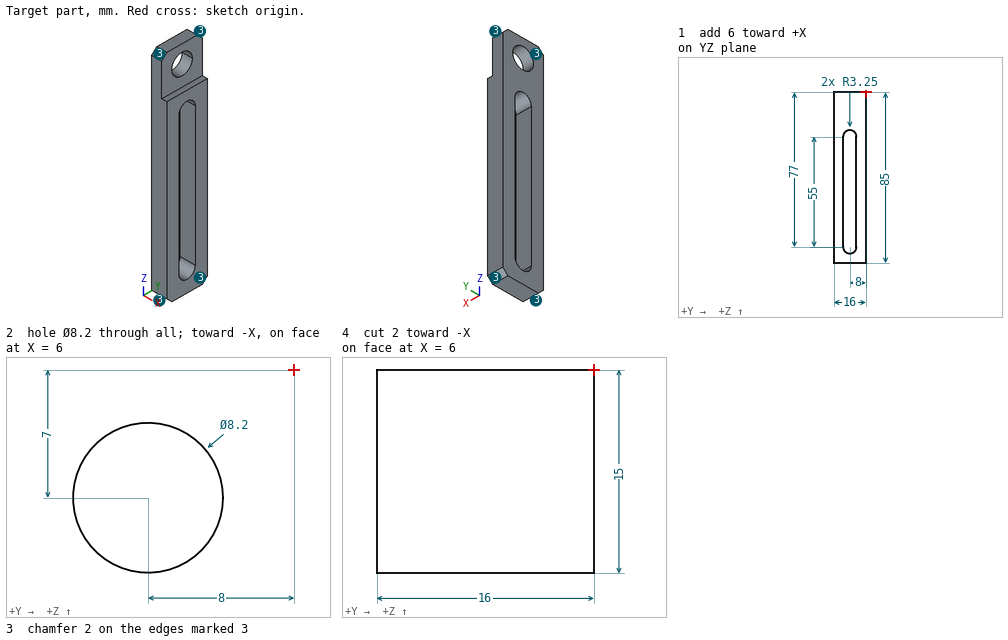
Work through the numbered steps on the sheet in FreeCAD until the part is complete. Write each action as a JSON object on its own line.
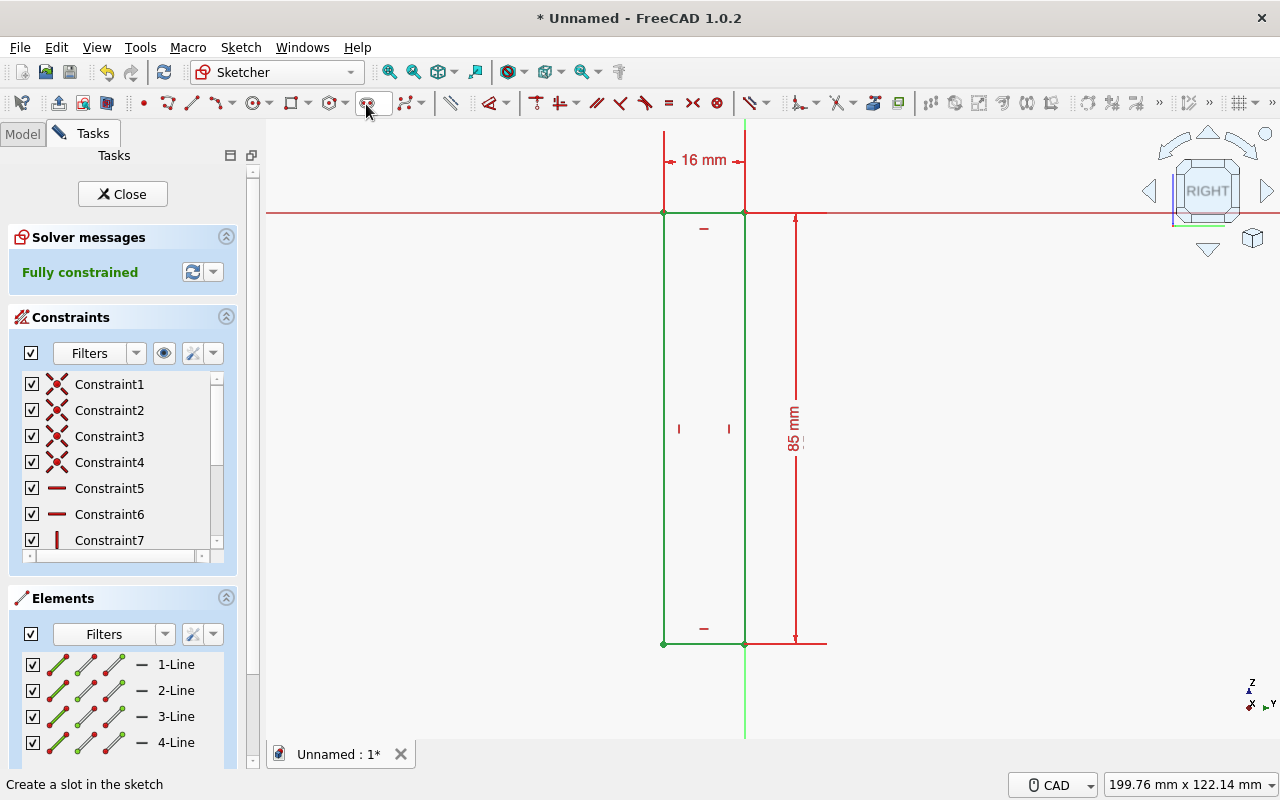
{"action": "scroll", "coordinate": [704, 604], "scroll_direction": "up", "scroll_amount": 2}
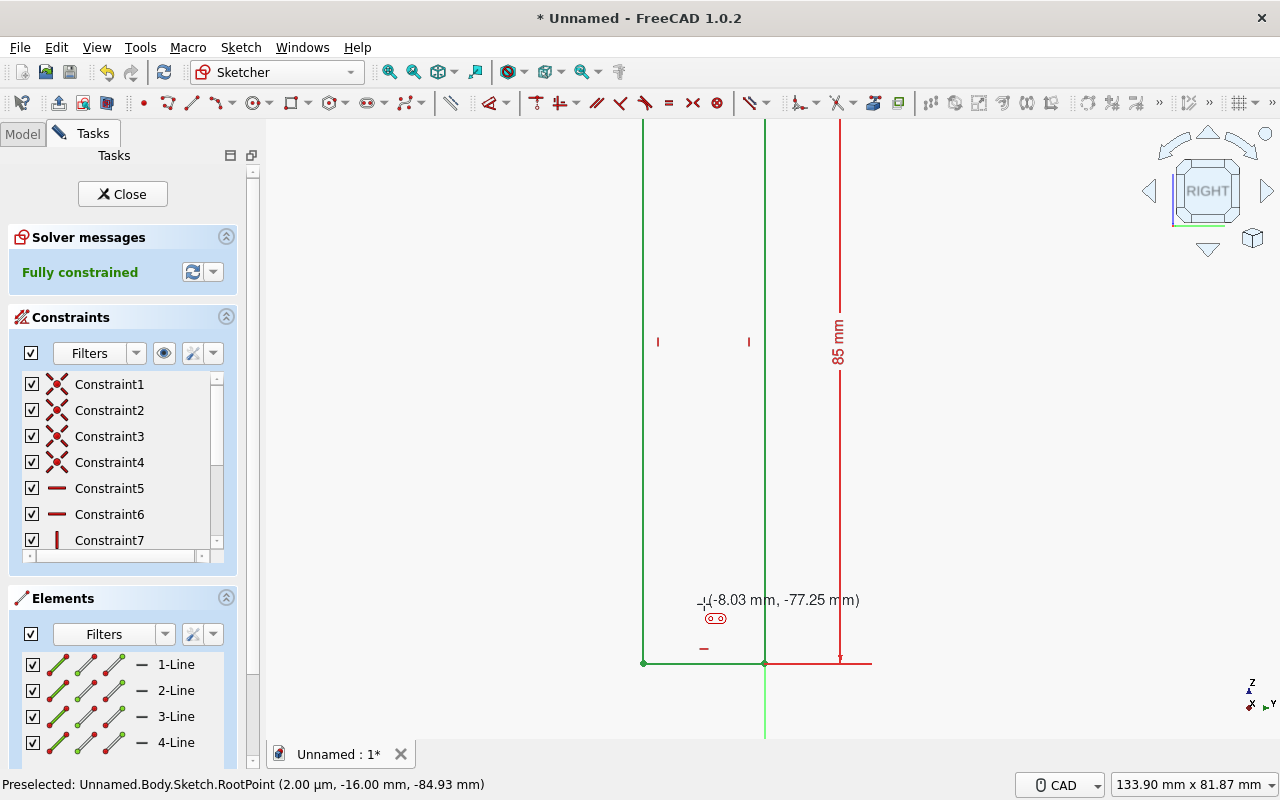
{"action": "left_click", "coordinate": [704, 603]}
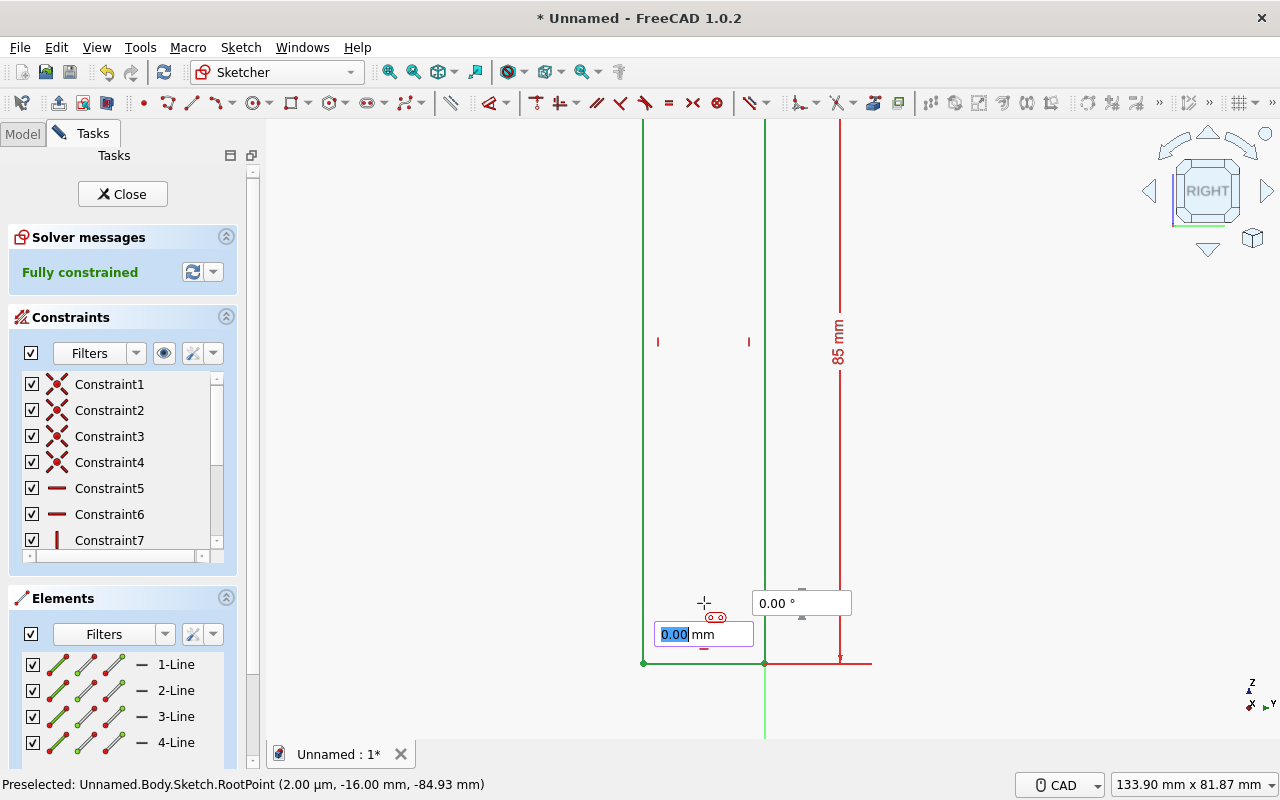
{"action": "left_click", "coordinate": [704, 187]}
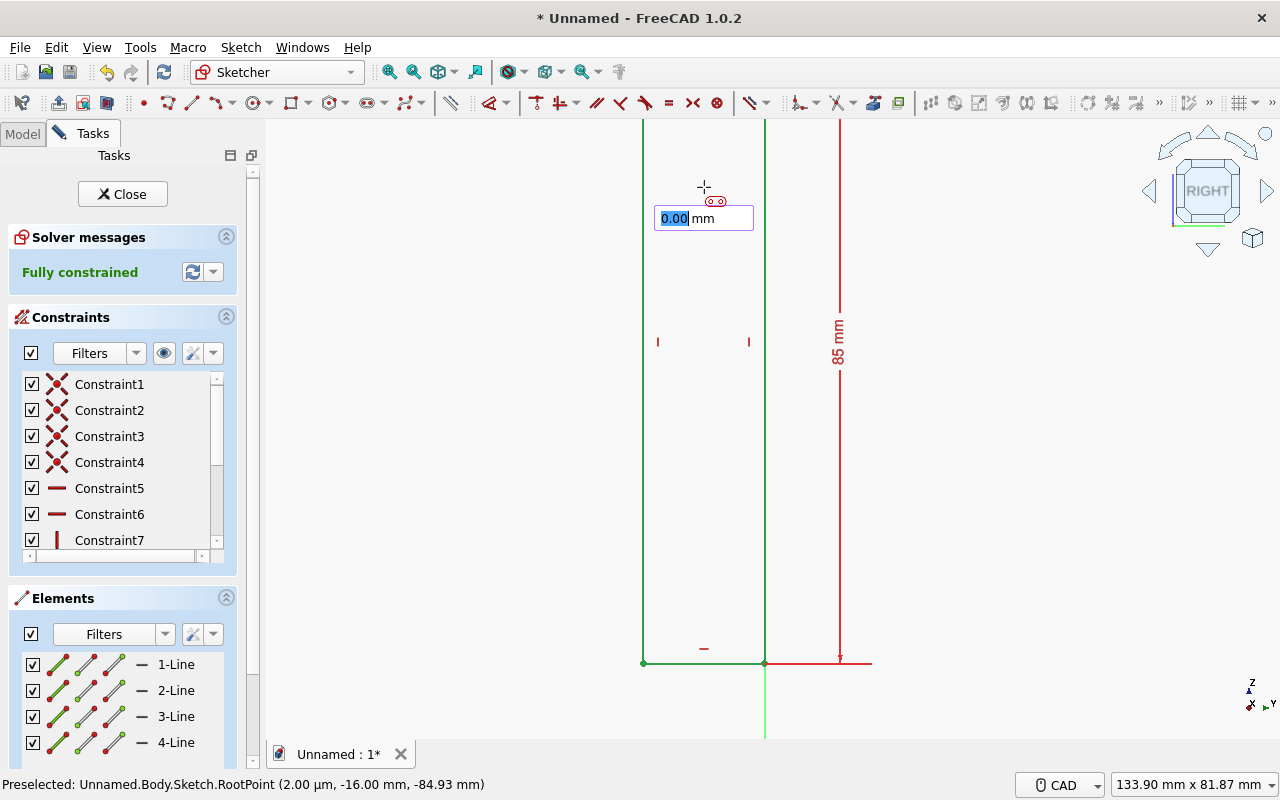
{"action": "left_click", "coordinate": [729, 395]}
{"action": "key", "text": "Escape"}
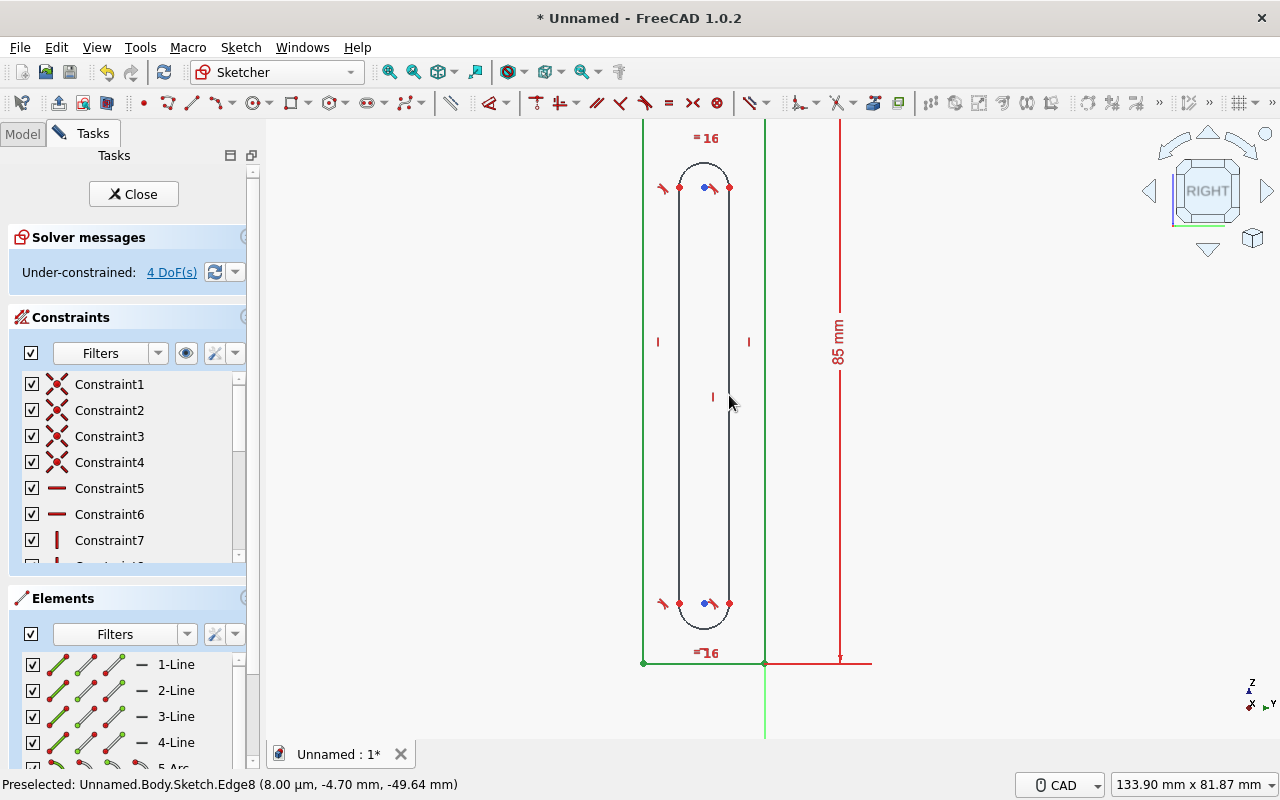
{"action": "left_click", "coordinate": [490, 104]}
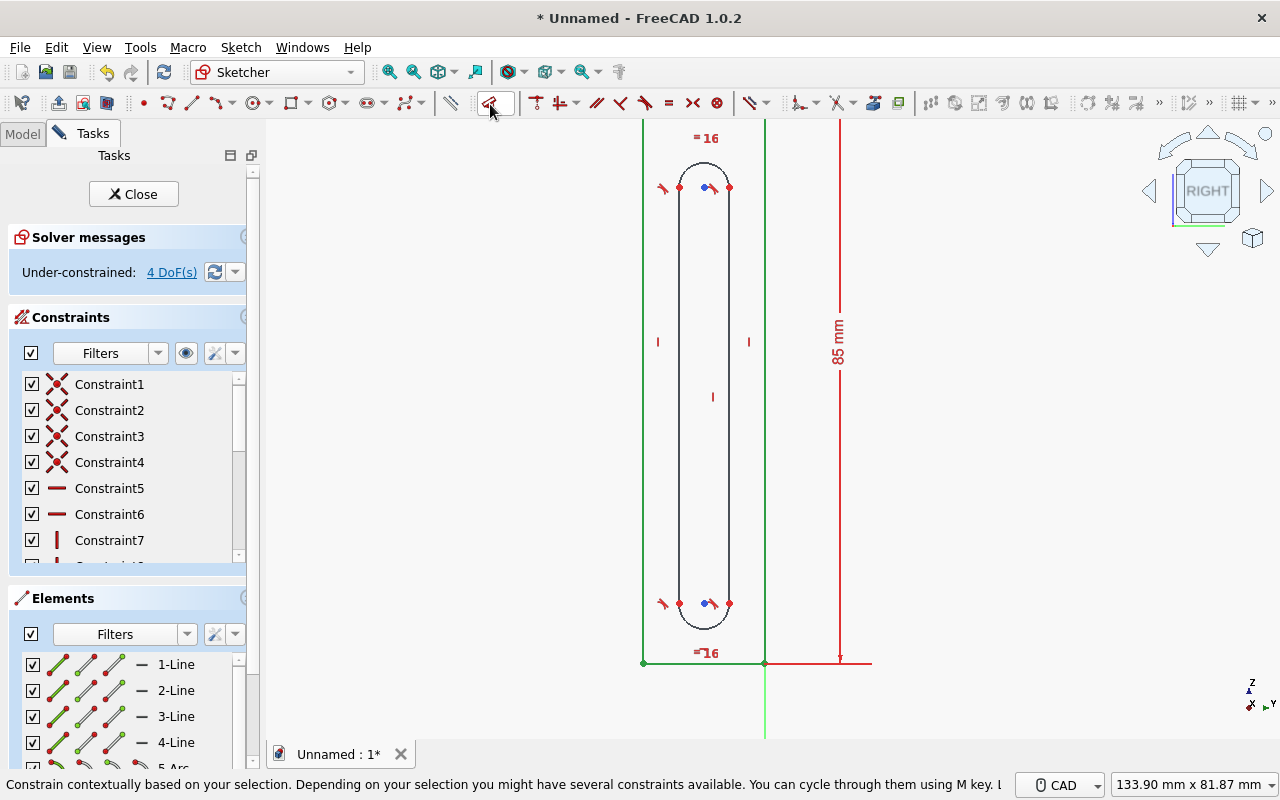
{"action": "scroll", "coordinate": [689, 624], "scroll_direction": "up", "scroll_amount": 3}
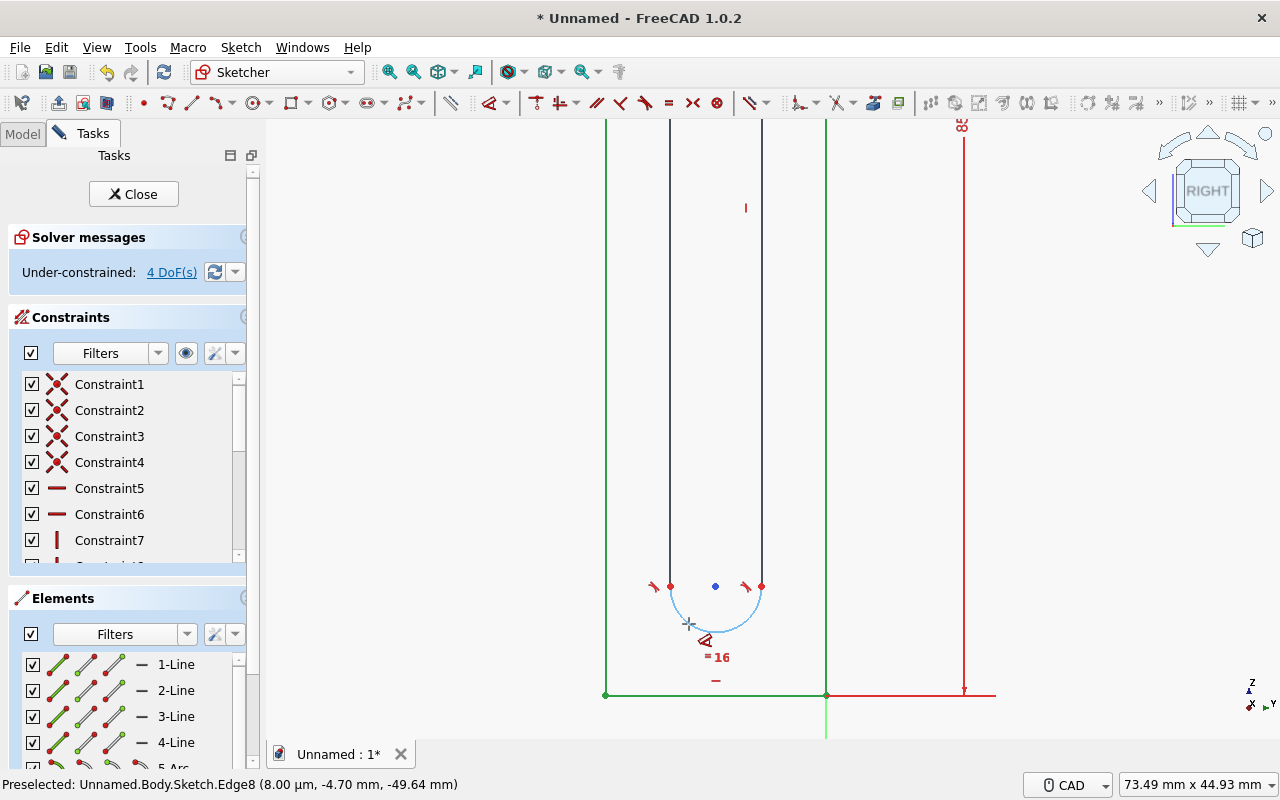
{"action": "left_click", "coordinate": [689, 624]}
{"action": "left_click", "coordinate": [670, 650]}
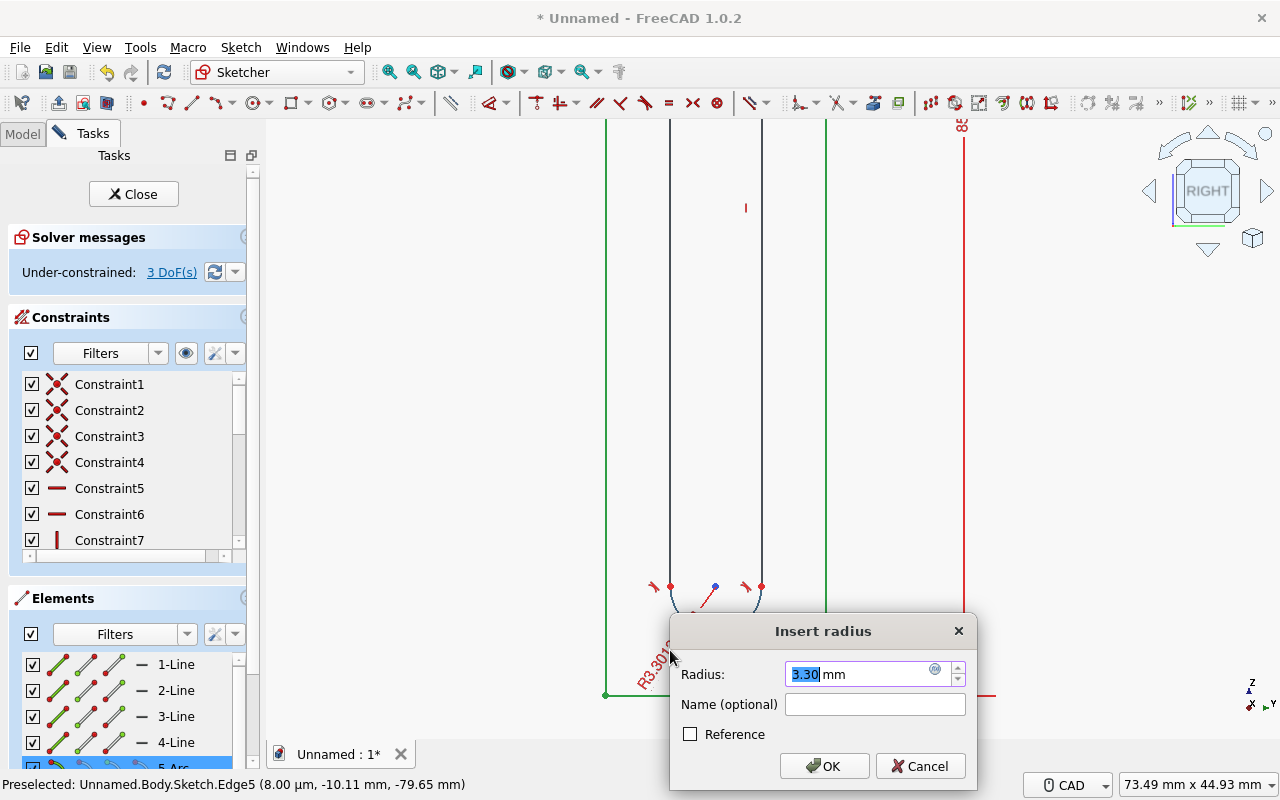
{"action": "type", "text": "3.25"}
{"action": "key", "text": "Return"}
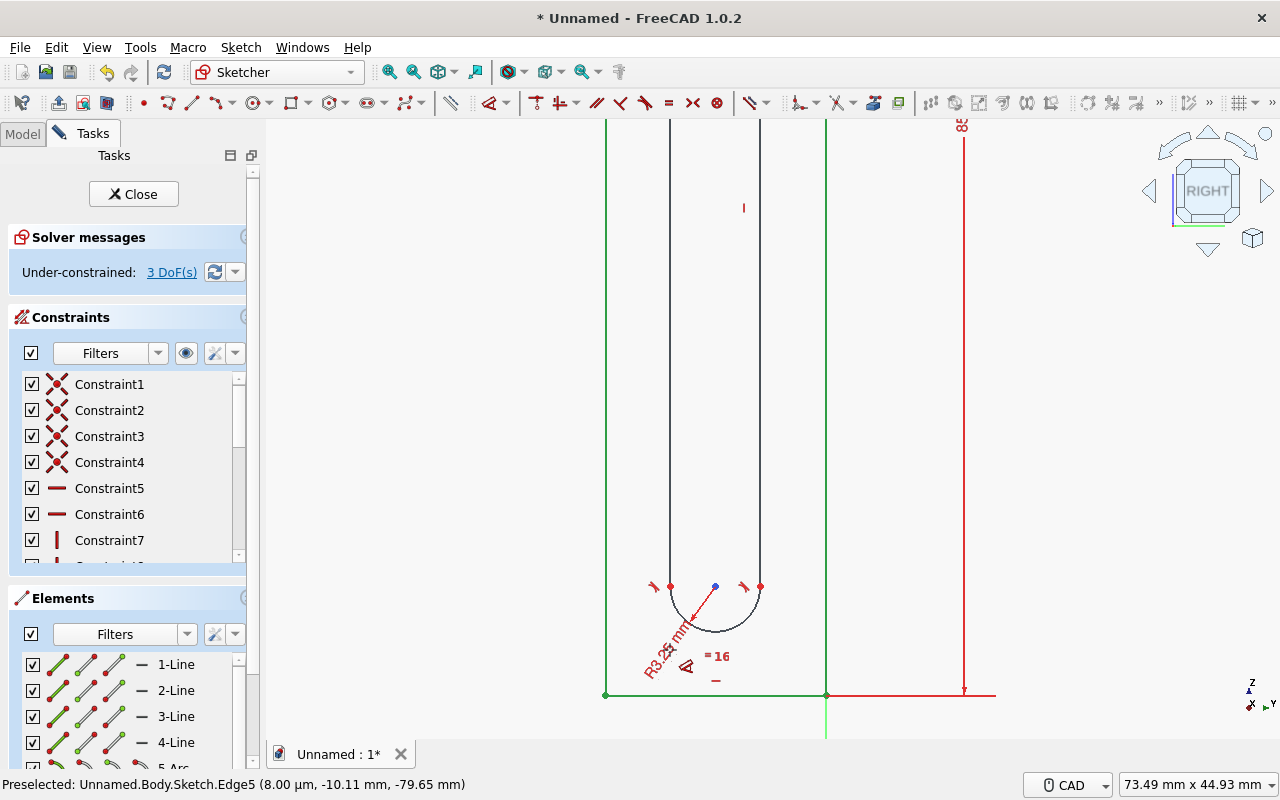
{"action": "left_click", "coordinate": [670, 359]}
{"action": "left_click", "coordinate": [636, 367]}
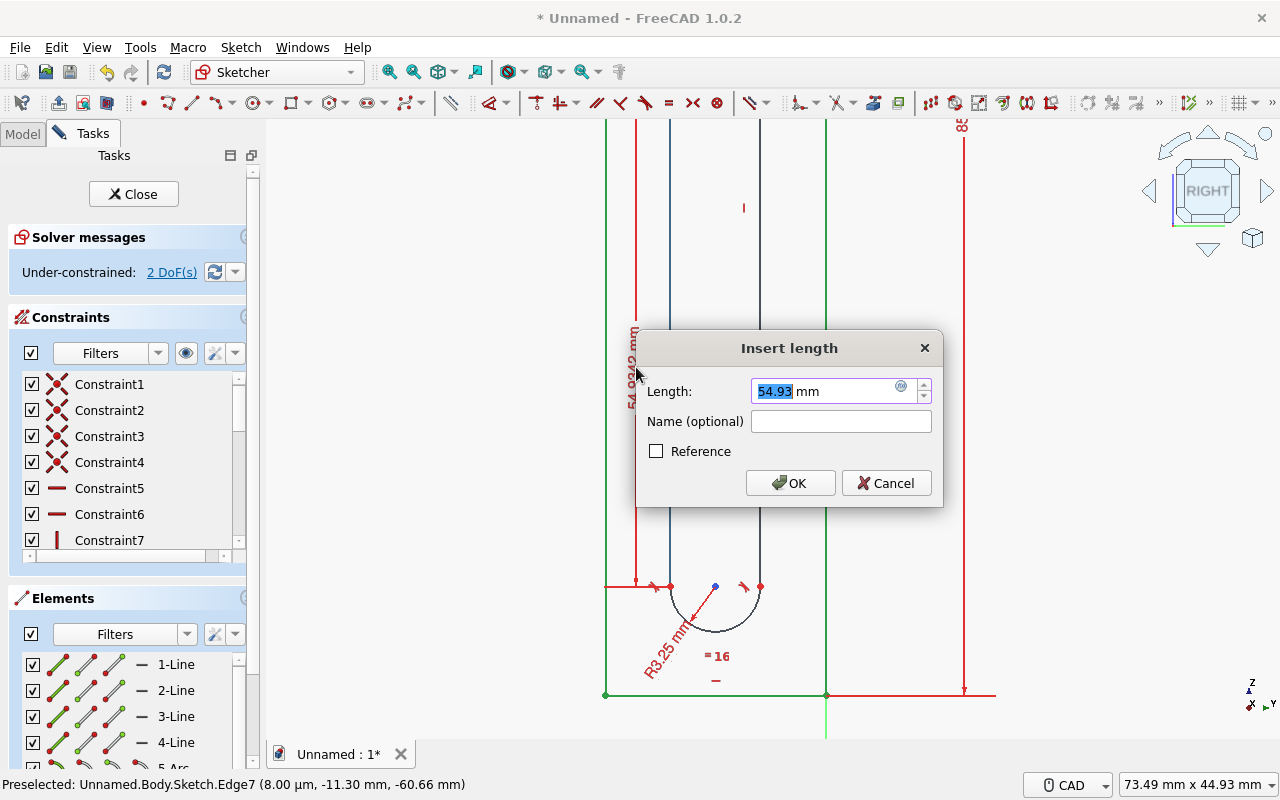
{"action": "type", "text": "55"}
{"action": "key", "text": "Return"}